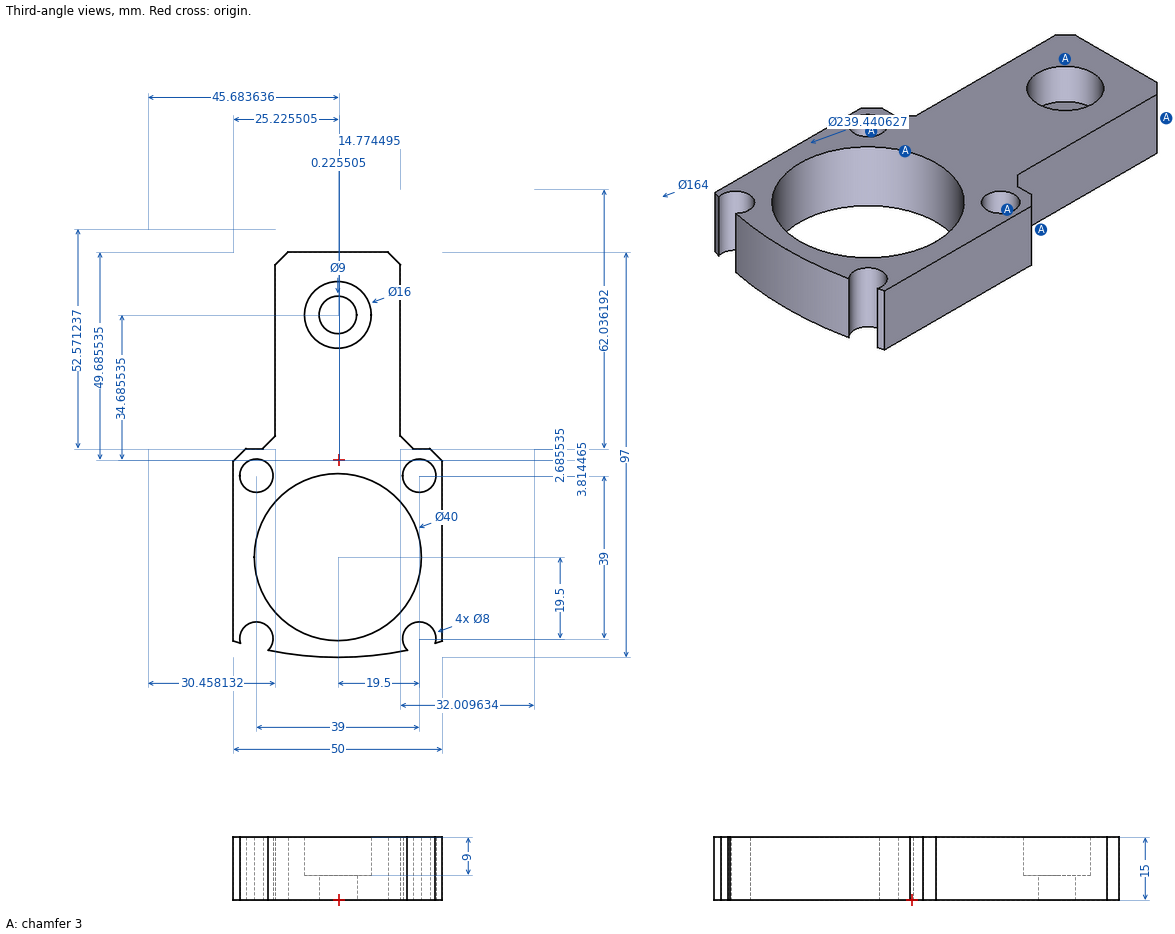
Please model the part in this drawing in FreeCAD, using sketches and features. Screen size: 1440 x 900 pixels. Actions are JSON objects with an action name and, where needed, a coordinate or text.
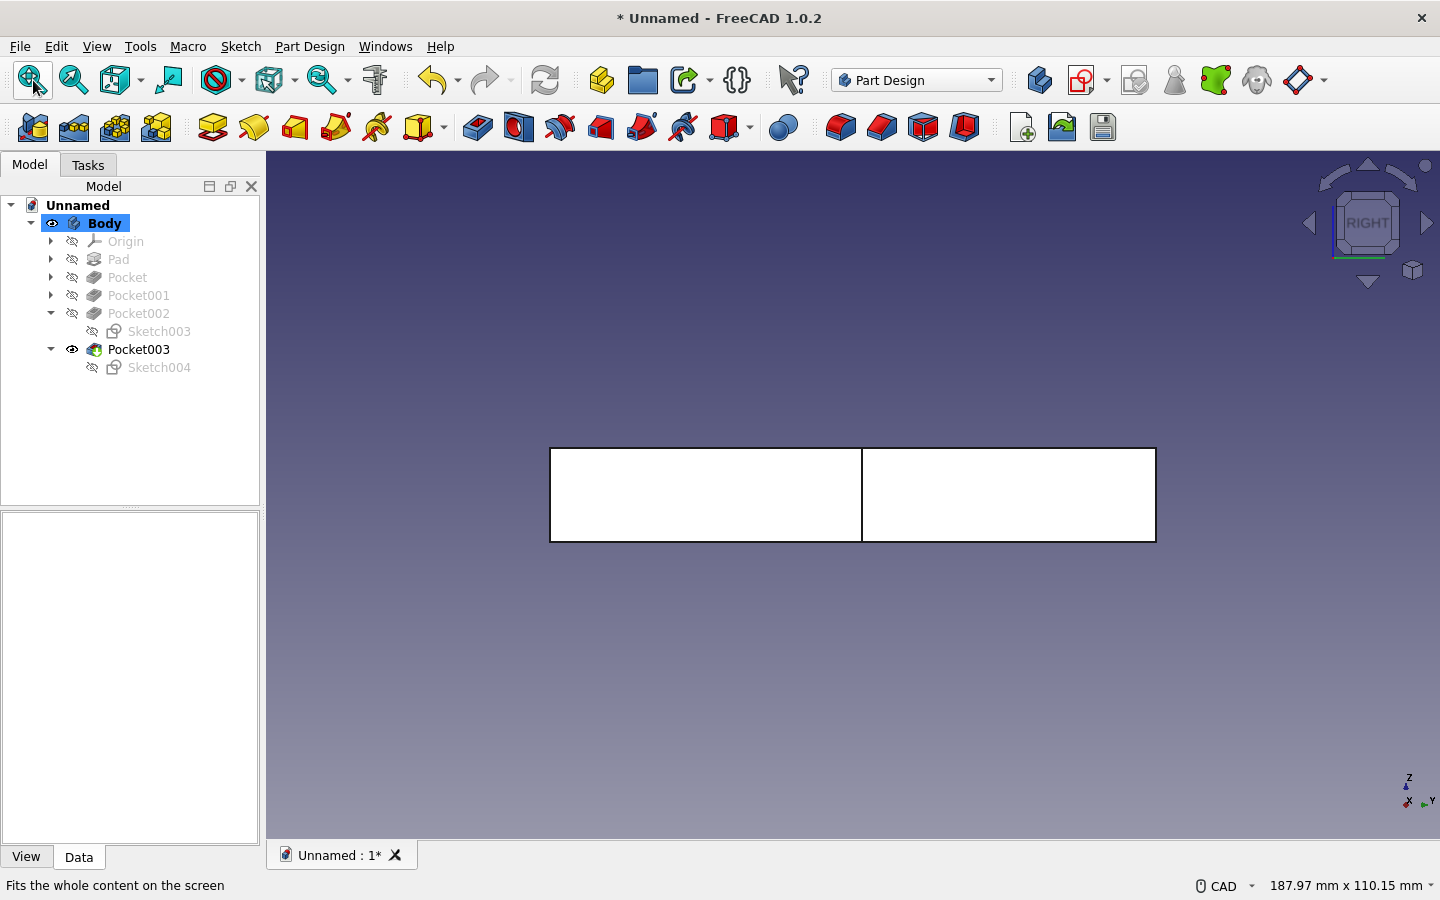
{"action": "left_click", "coordinate": [1156, 494]}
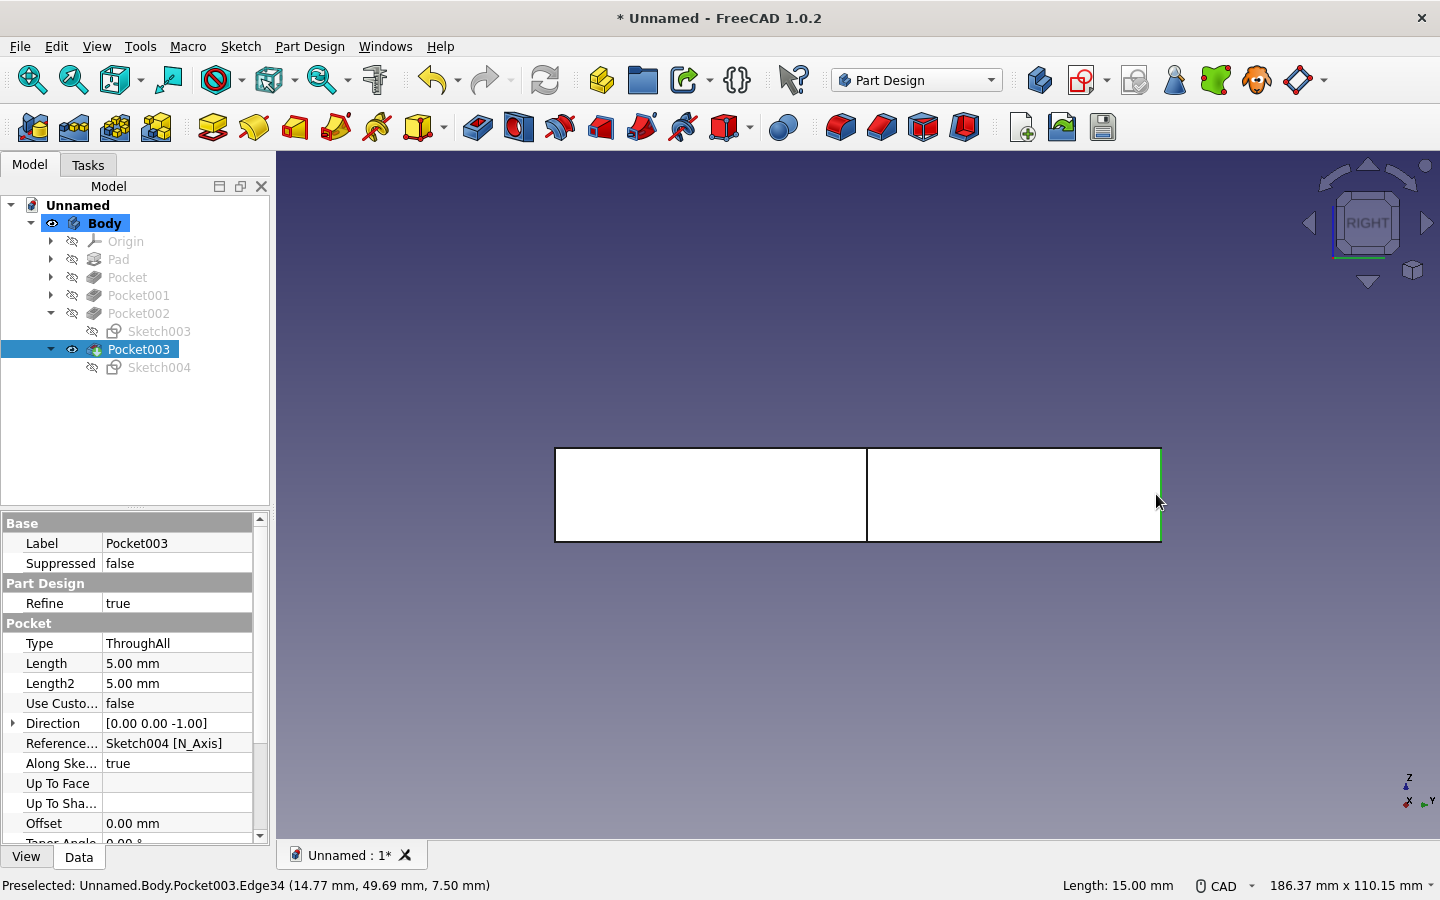
{"action": "left_click", "coordinate": [867, 494], "text": "ctrl"}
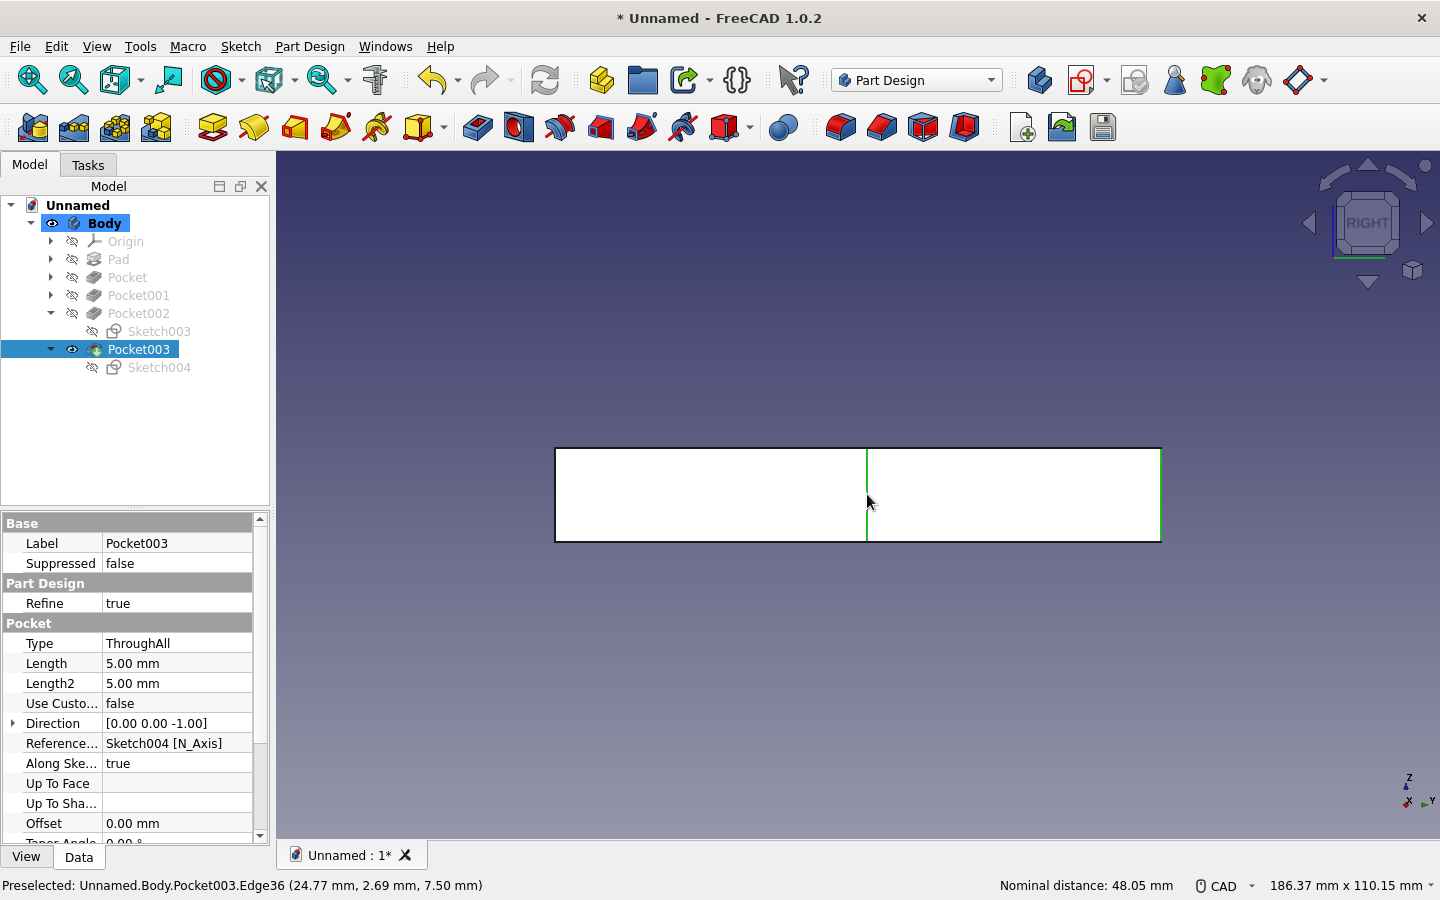
{"action": "key", "text": "5"}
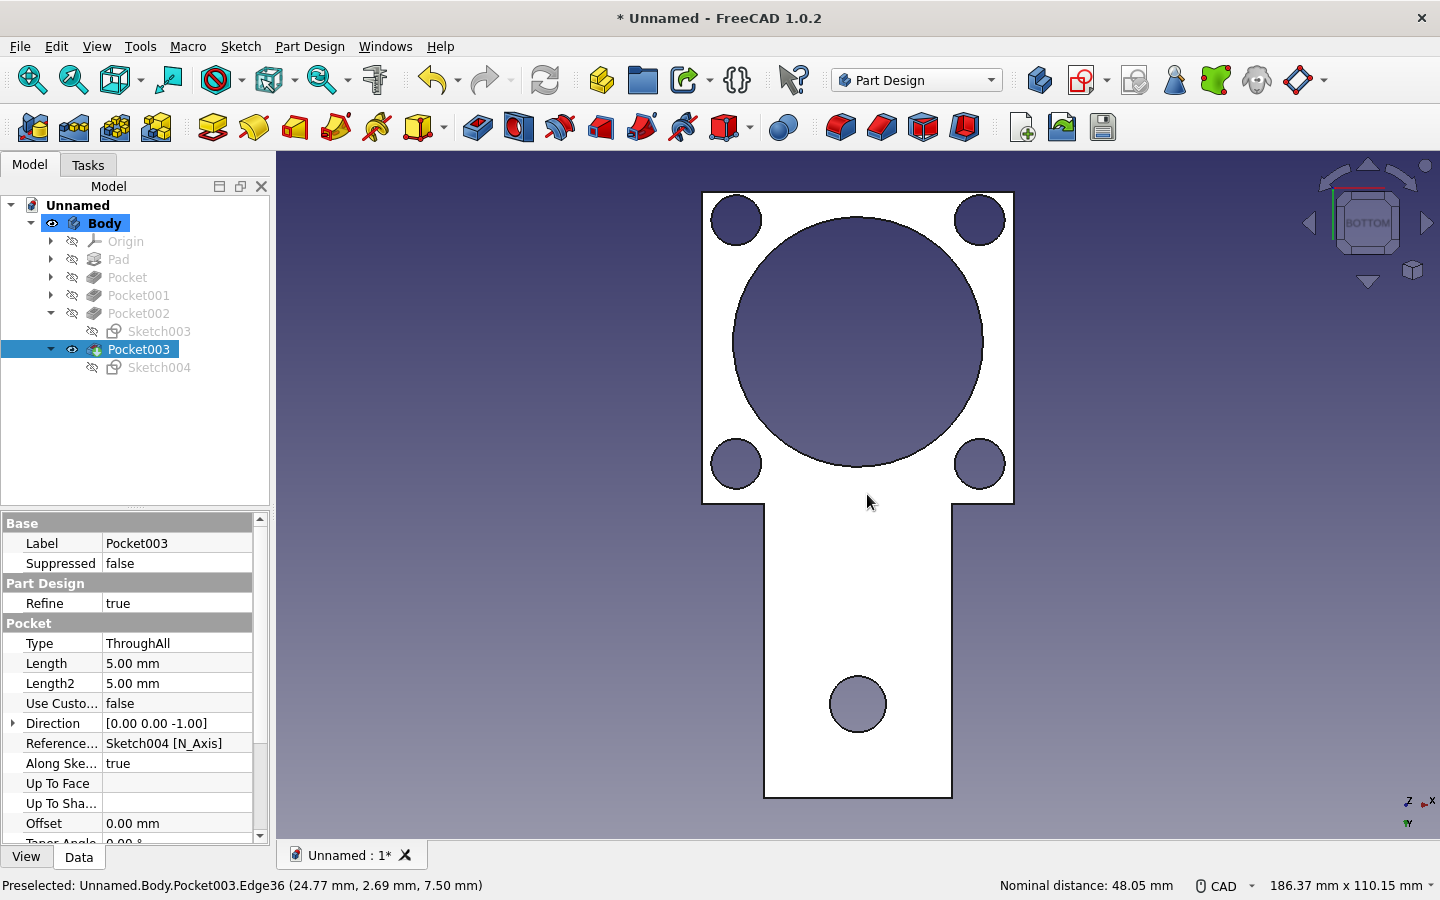
{"action": "key", "text": "4"}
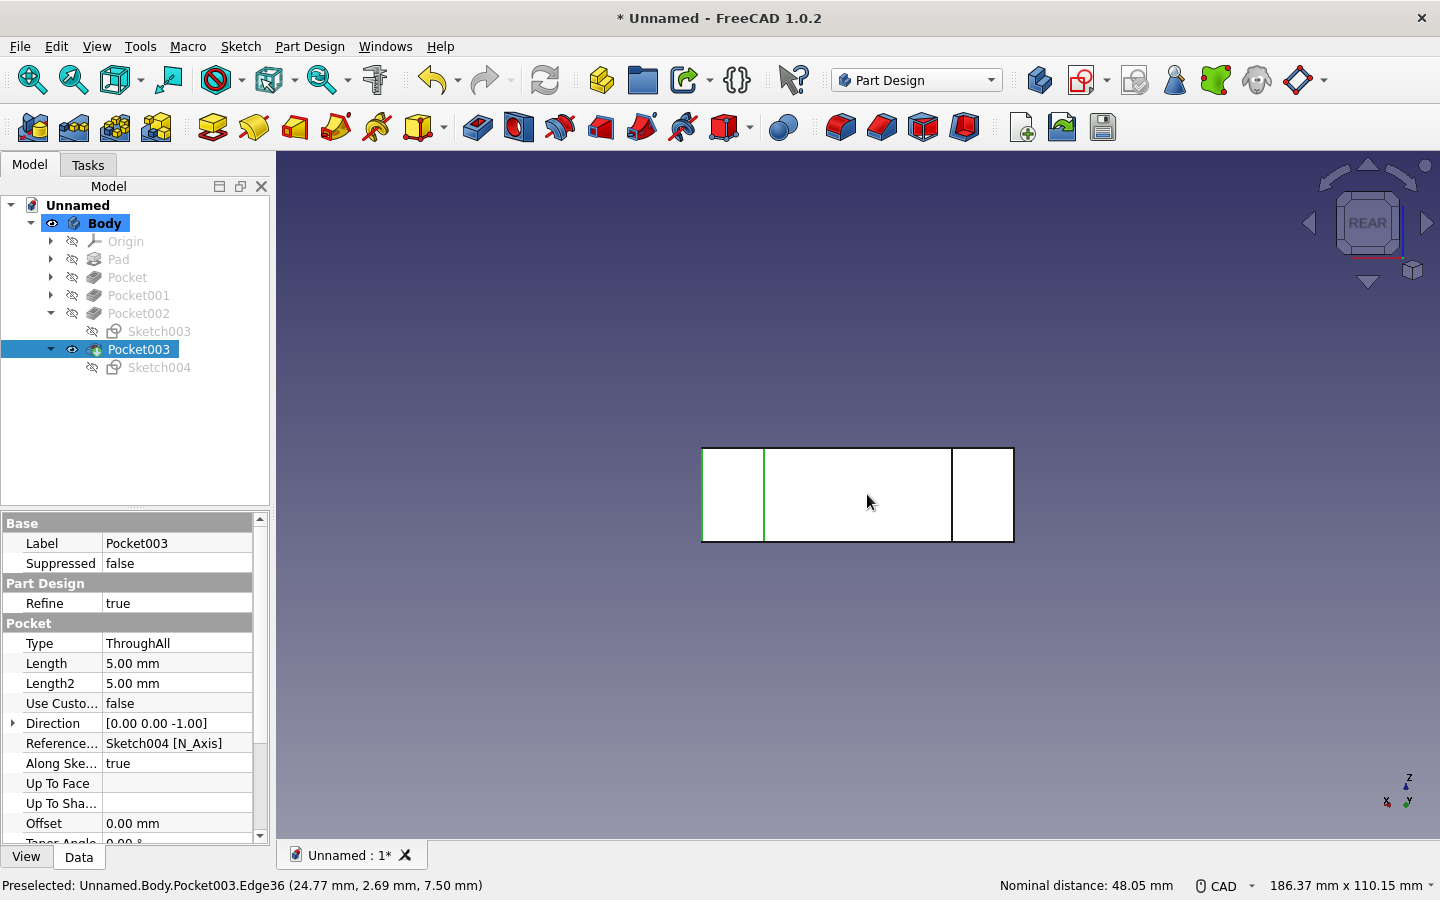
{"action": "left_click", "coordinate": [33, 80]}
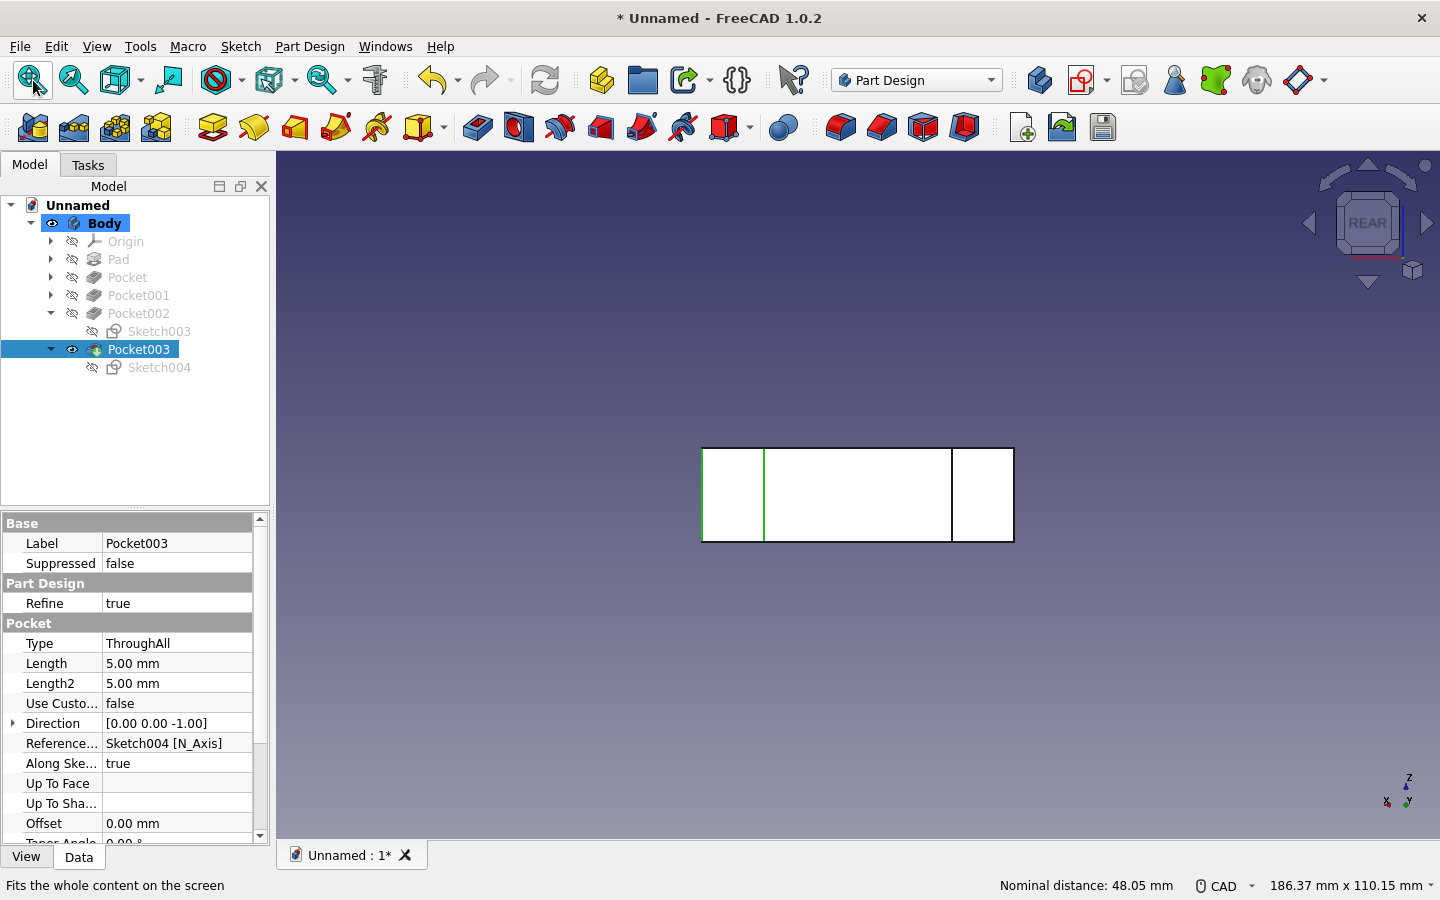
{"action": "left_click", "coordinate": [952, 494], "text": "ctrl"}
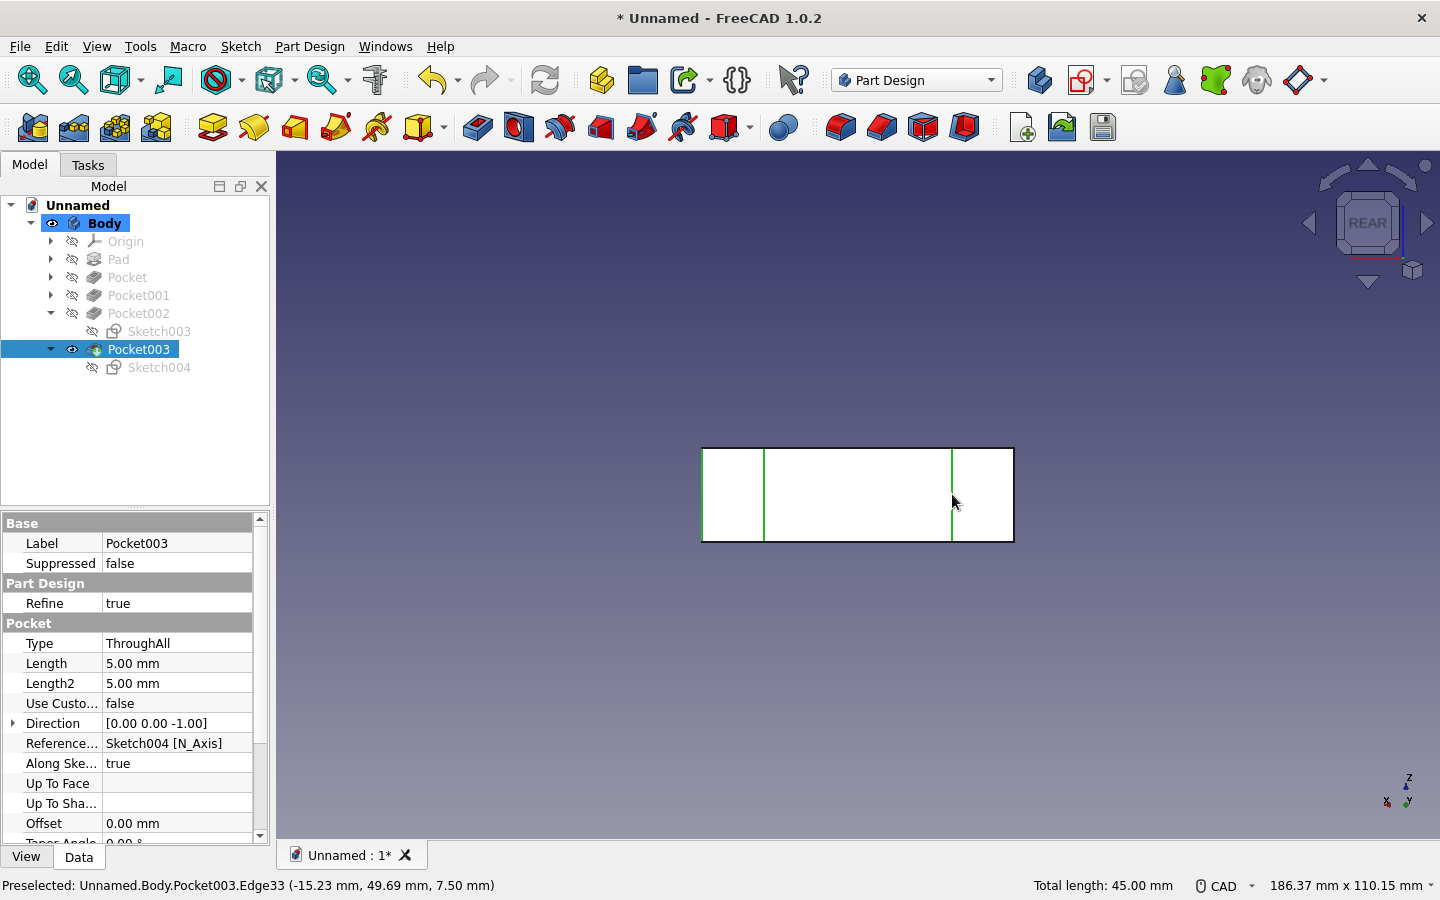
{"action": "left_click", "coordinate": [1014, 494], "text": "ctrl"}